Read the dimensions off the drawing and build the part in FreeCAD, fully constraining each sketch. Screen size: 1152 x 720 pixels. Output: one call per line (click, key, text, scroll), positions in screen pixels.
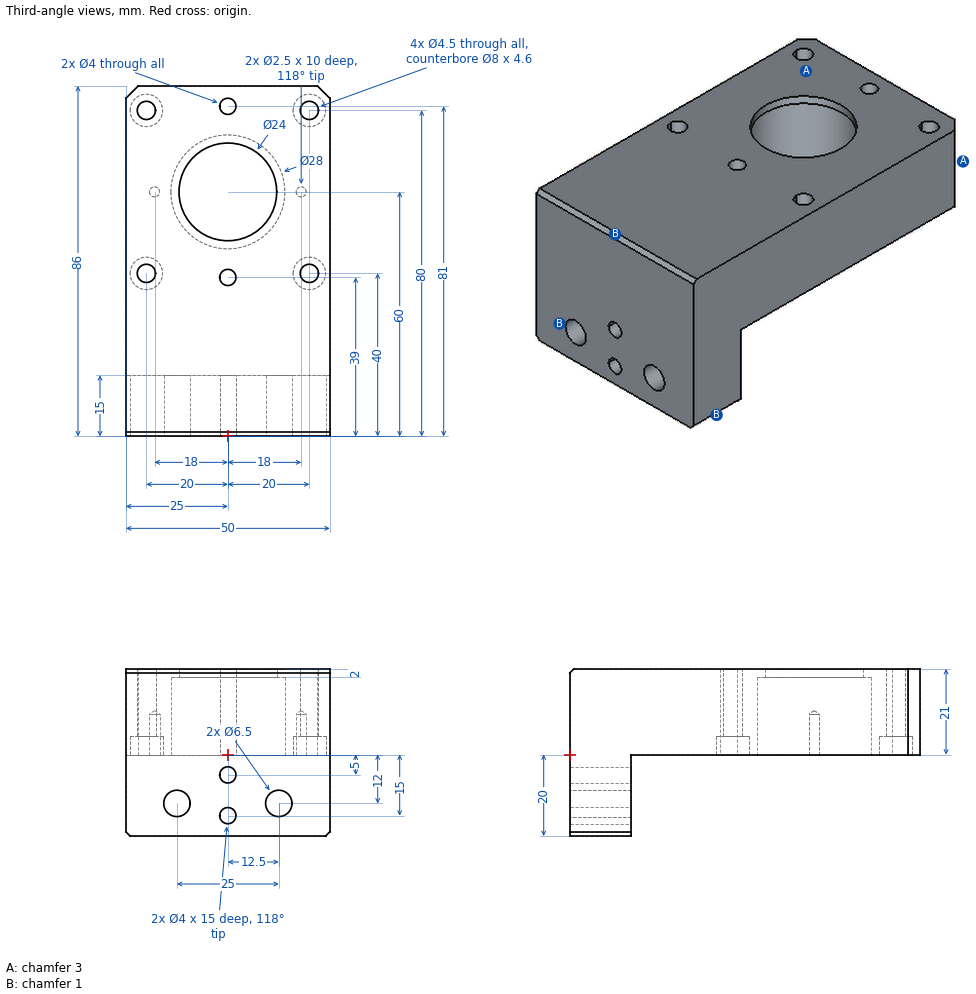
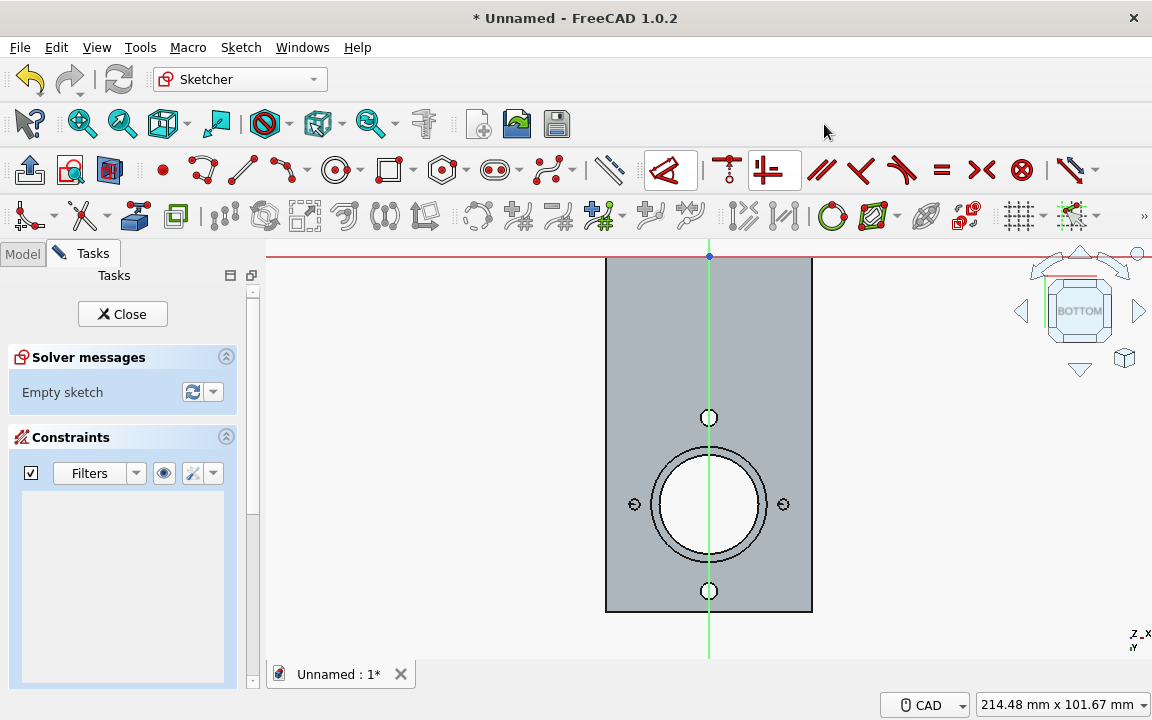
scroll(640, 449, down, 5)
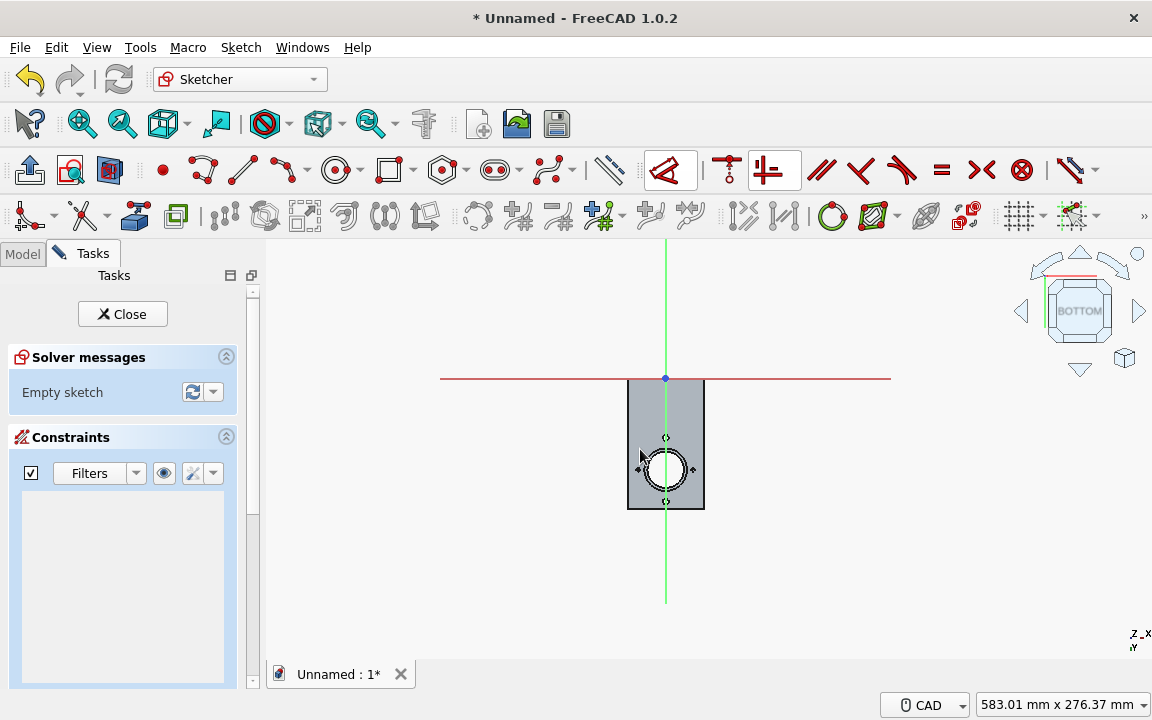
scroll(671, 378, up, 9)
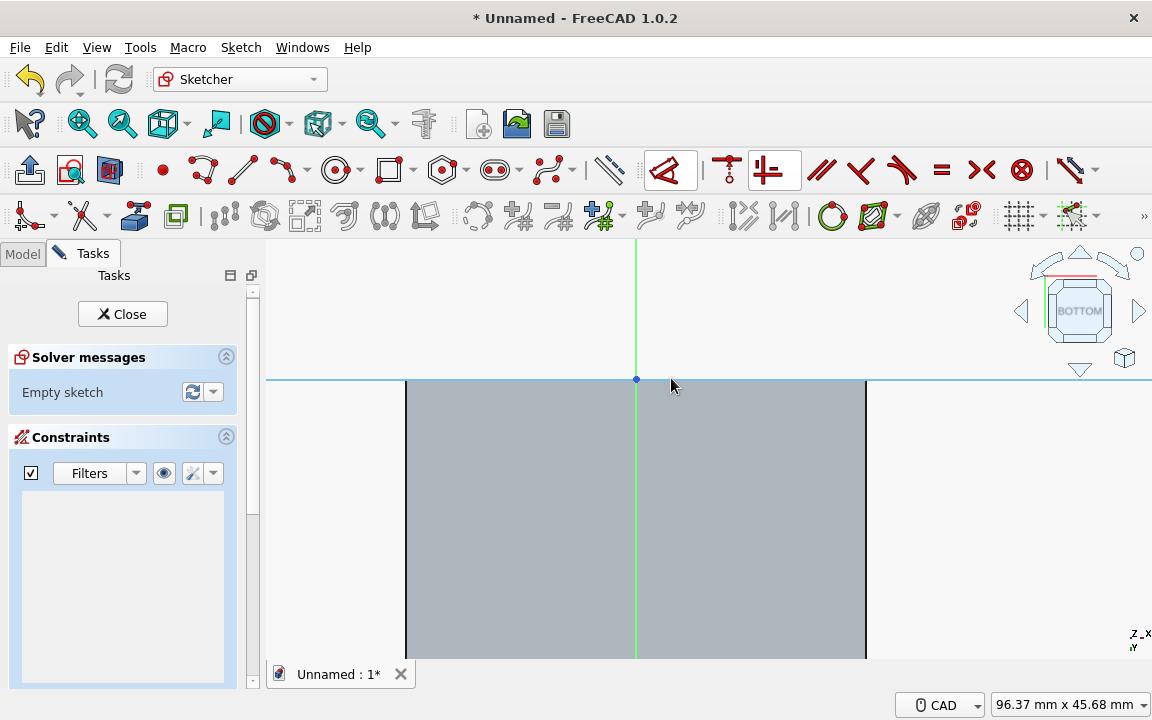
key(g)
key(r)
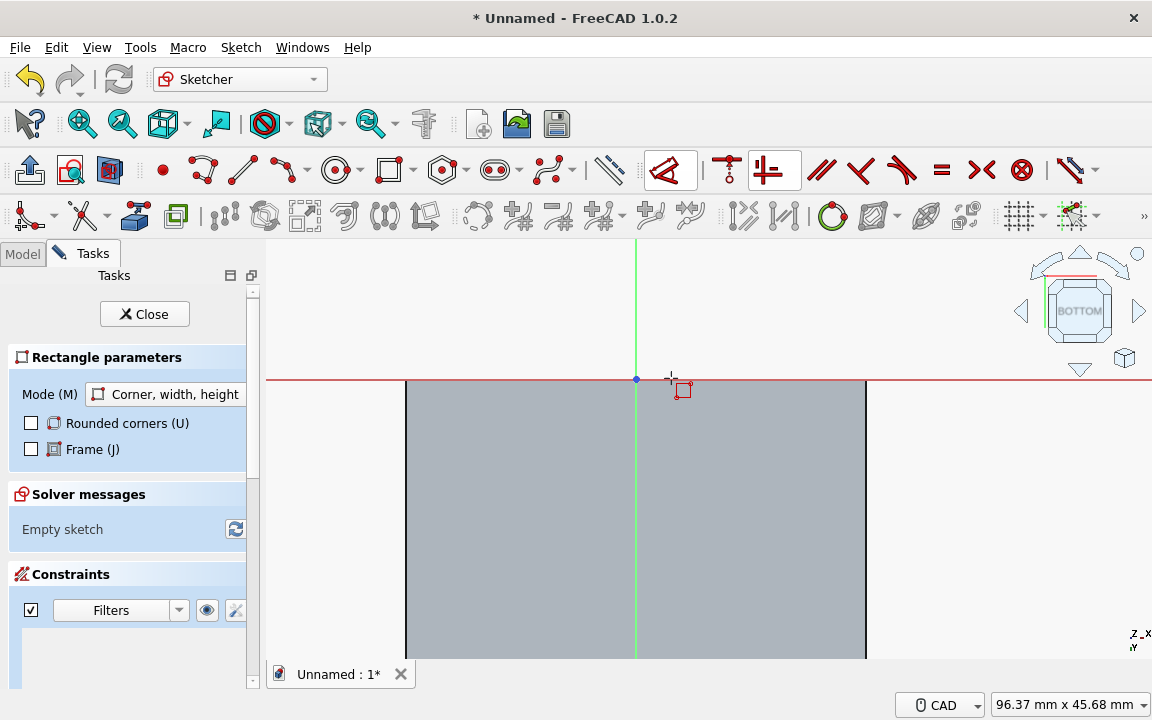
click(406, 380)
click(866, 518)
key(Escape)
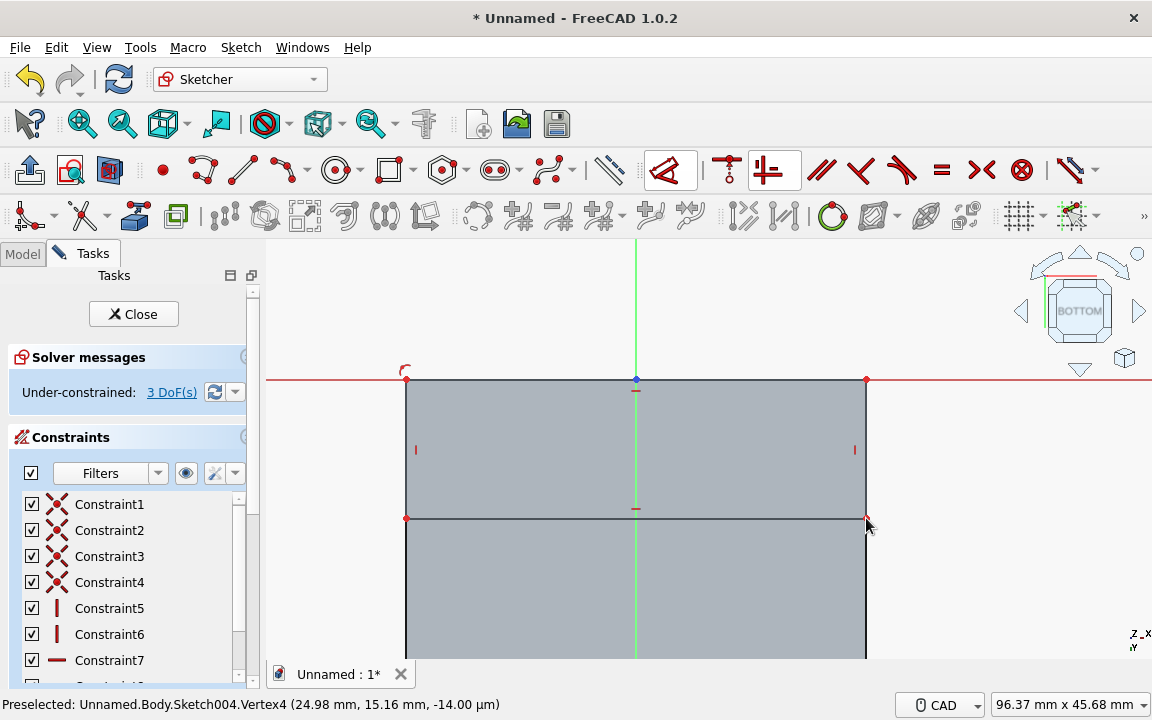
click(406, 421)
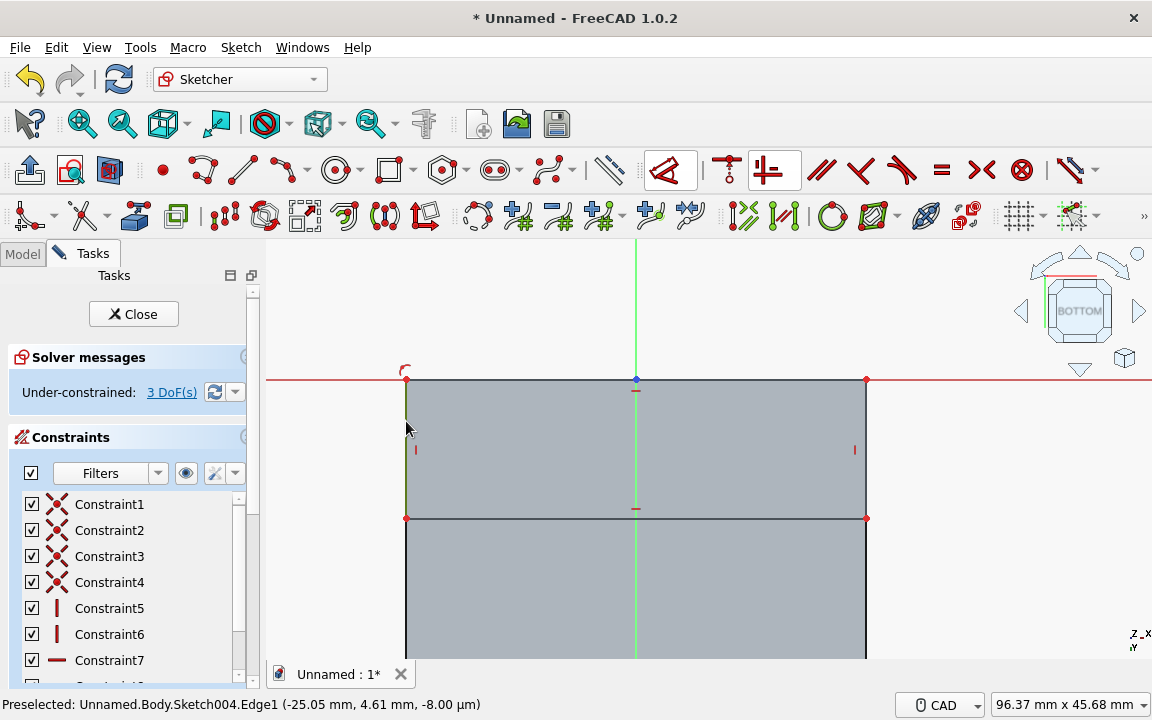
click(692, 170)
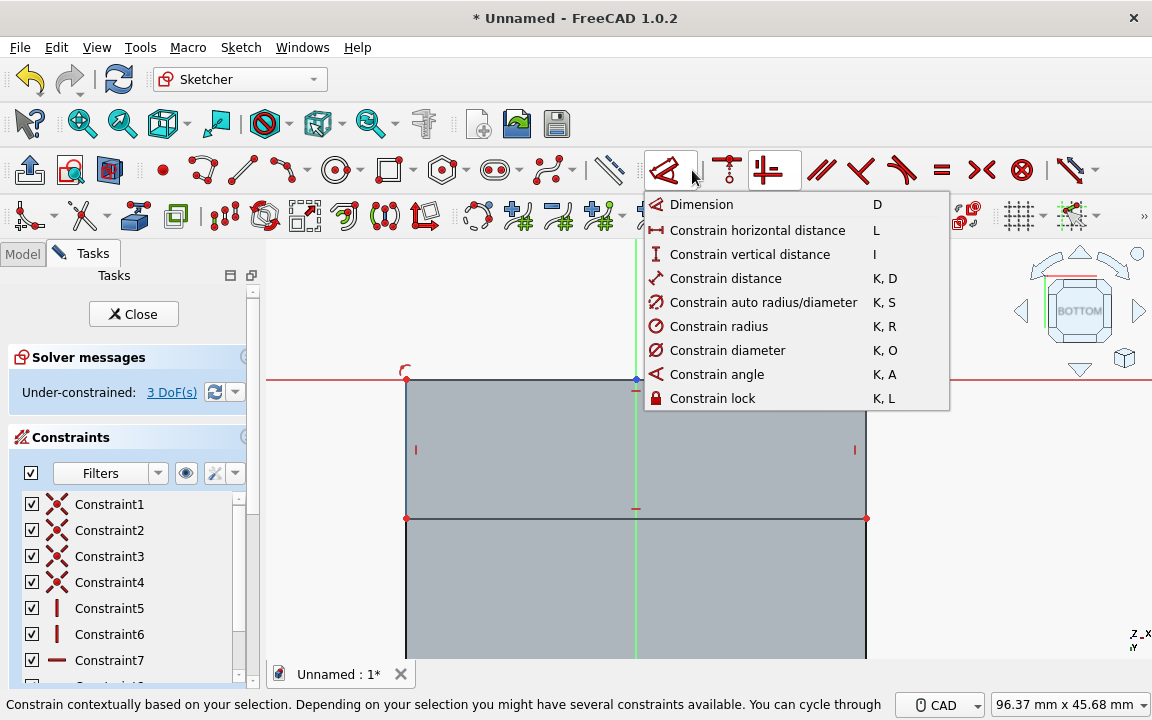
click(797, 254)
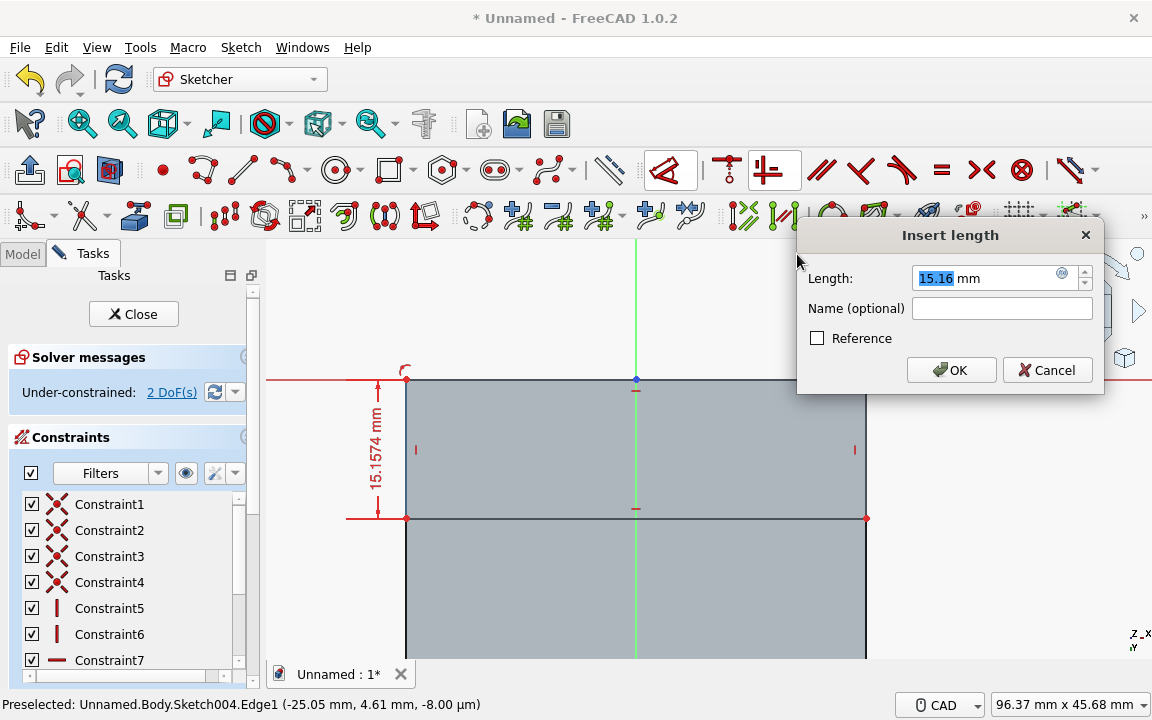
text(15)
key(Return)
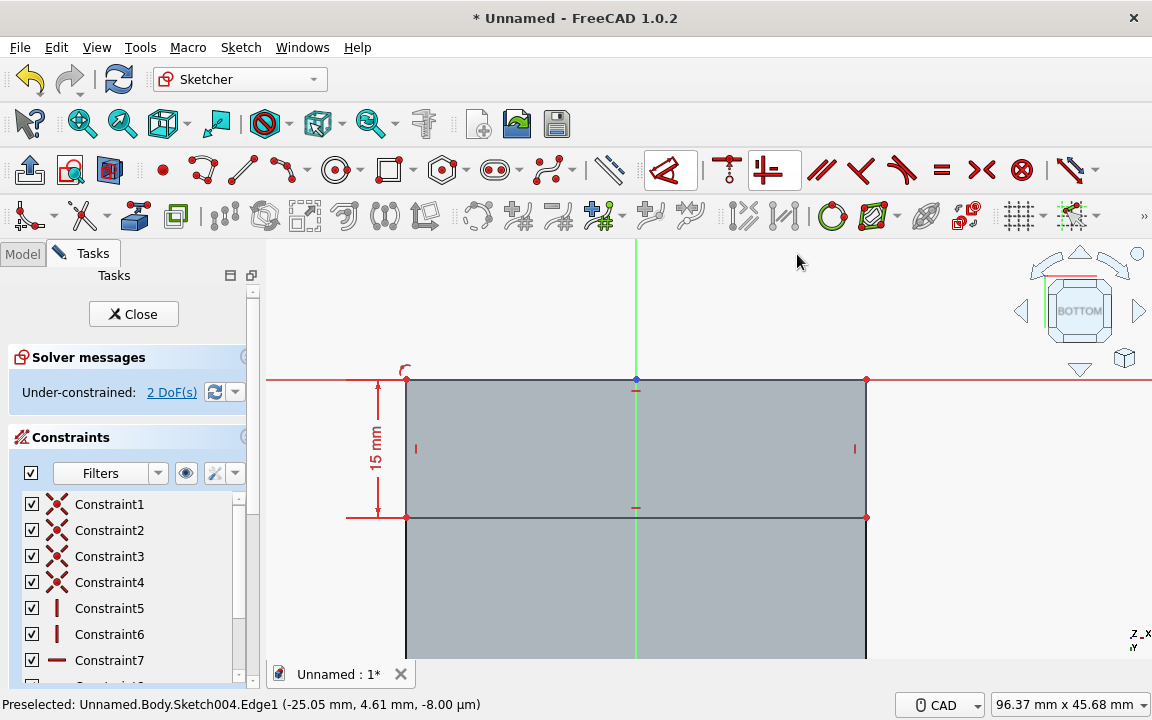
click(544, 518)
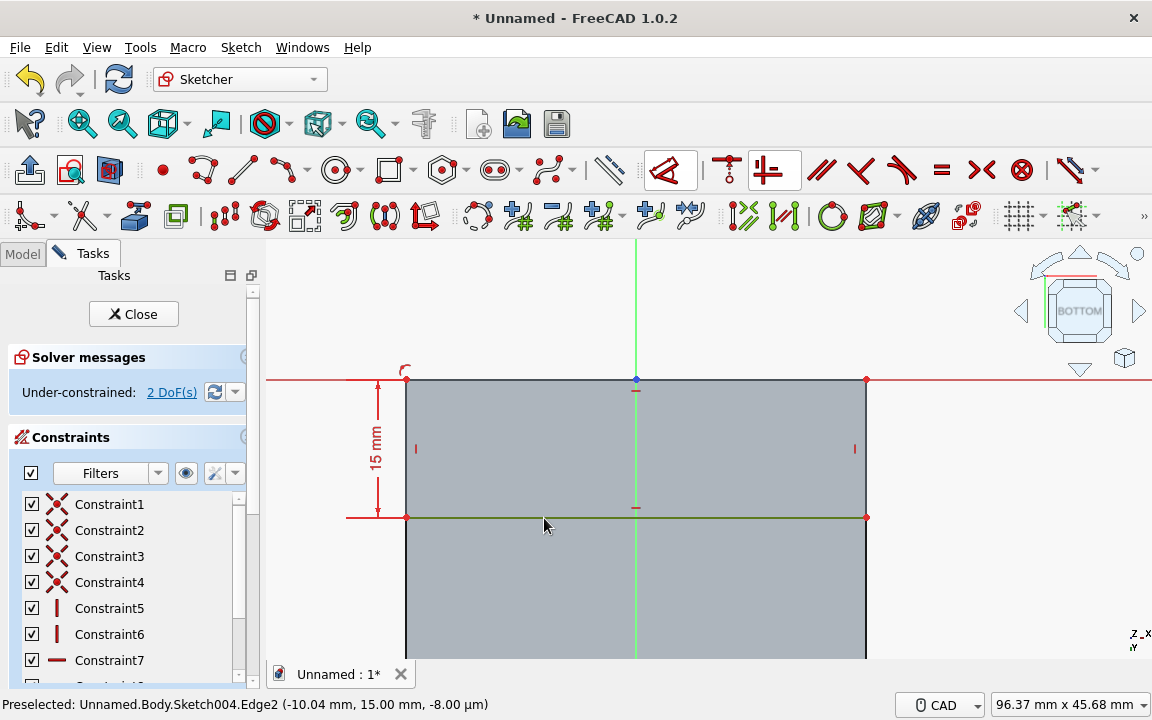
click(692, 170)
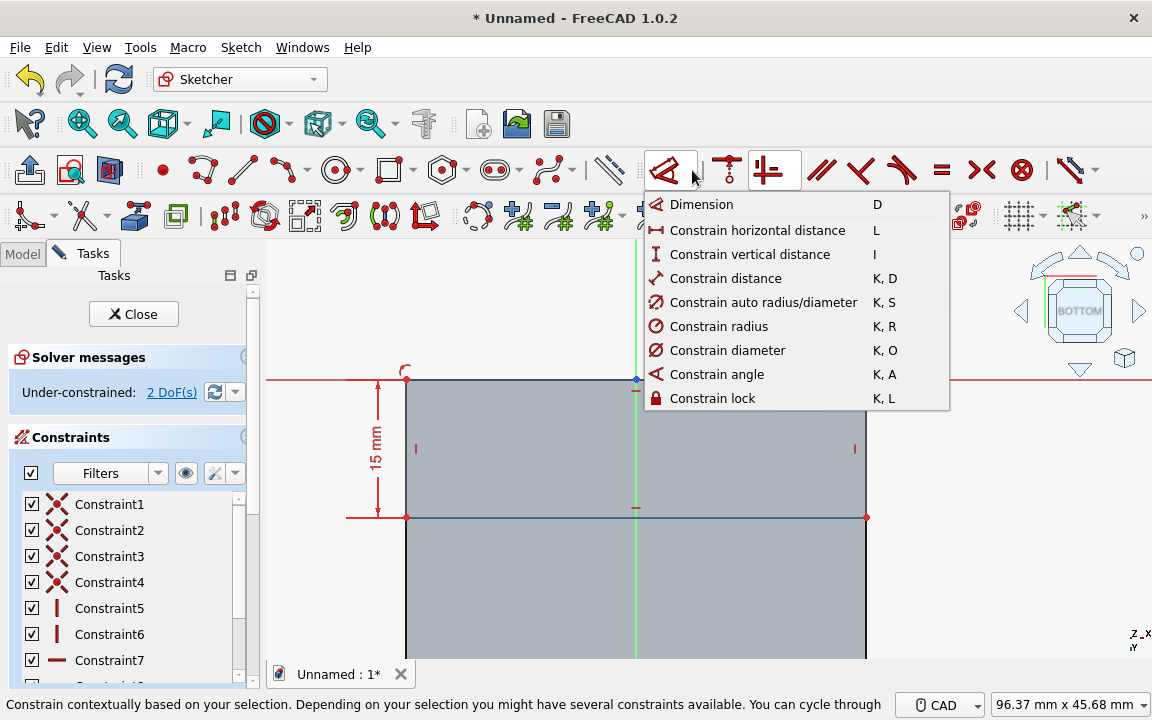
click(797, 230)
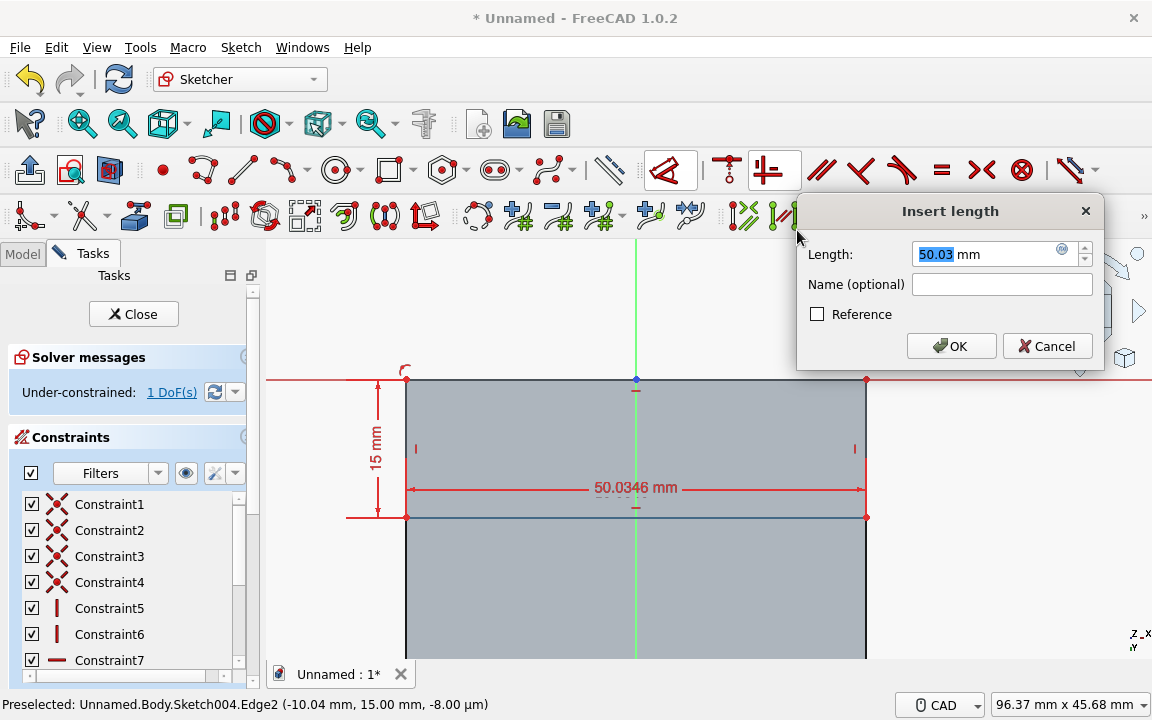
text(50)
key(Return)